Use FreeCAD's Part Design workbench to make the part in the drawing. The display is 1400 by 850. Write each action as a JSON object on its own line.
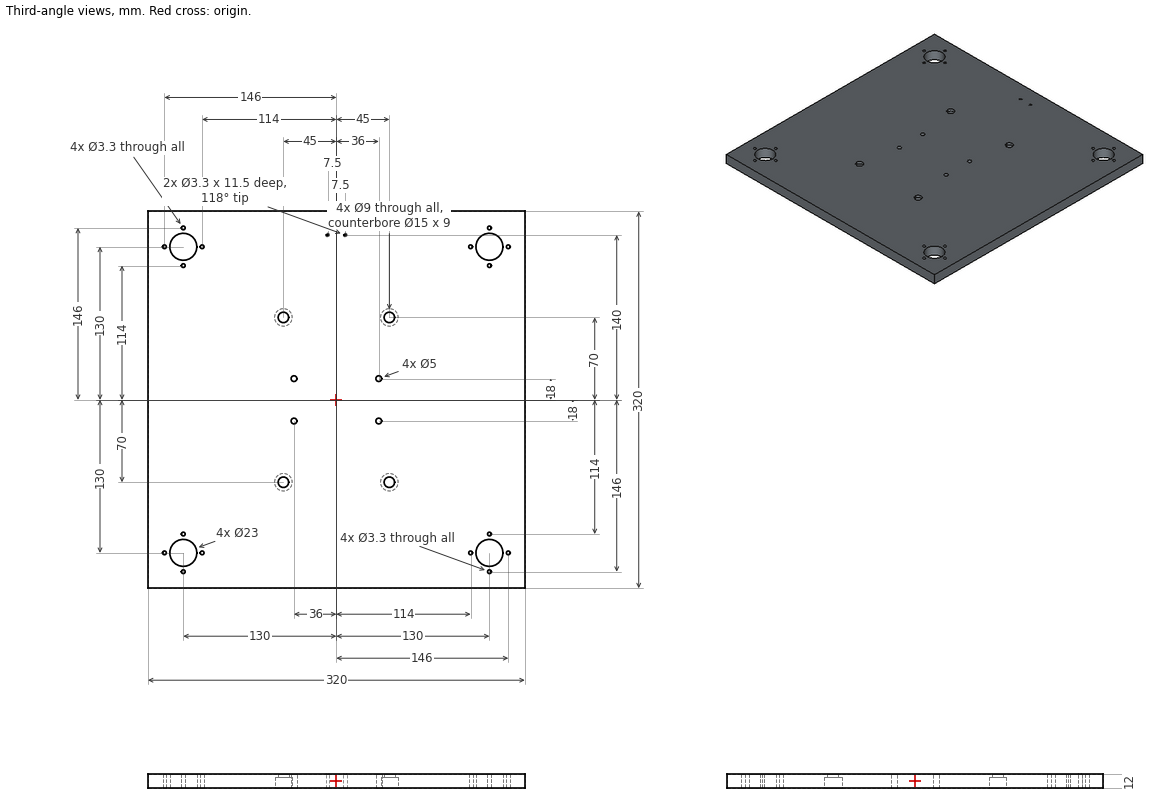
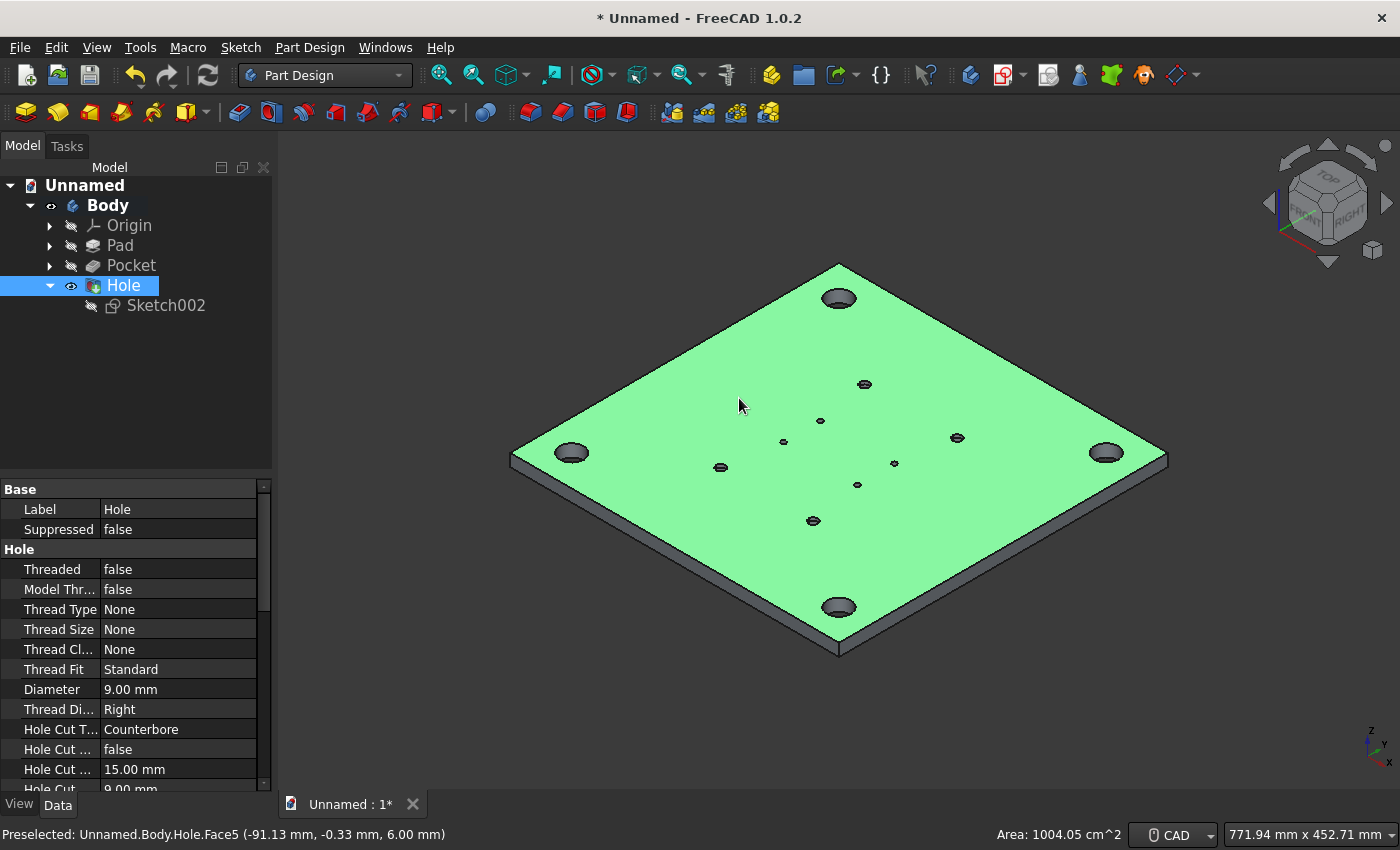
{"action": "left_click", "coordinate": [1004, 76]}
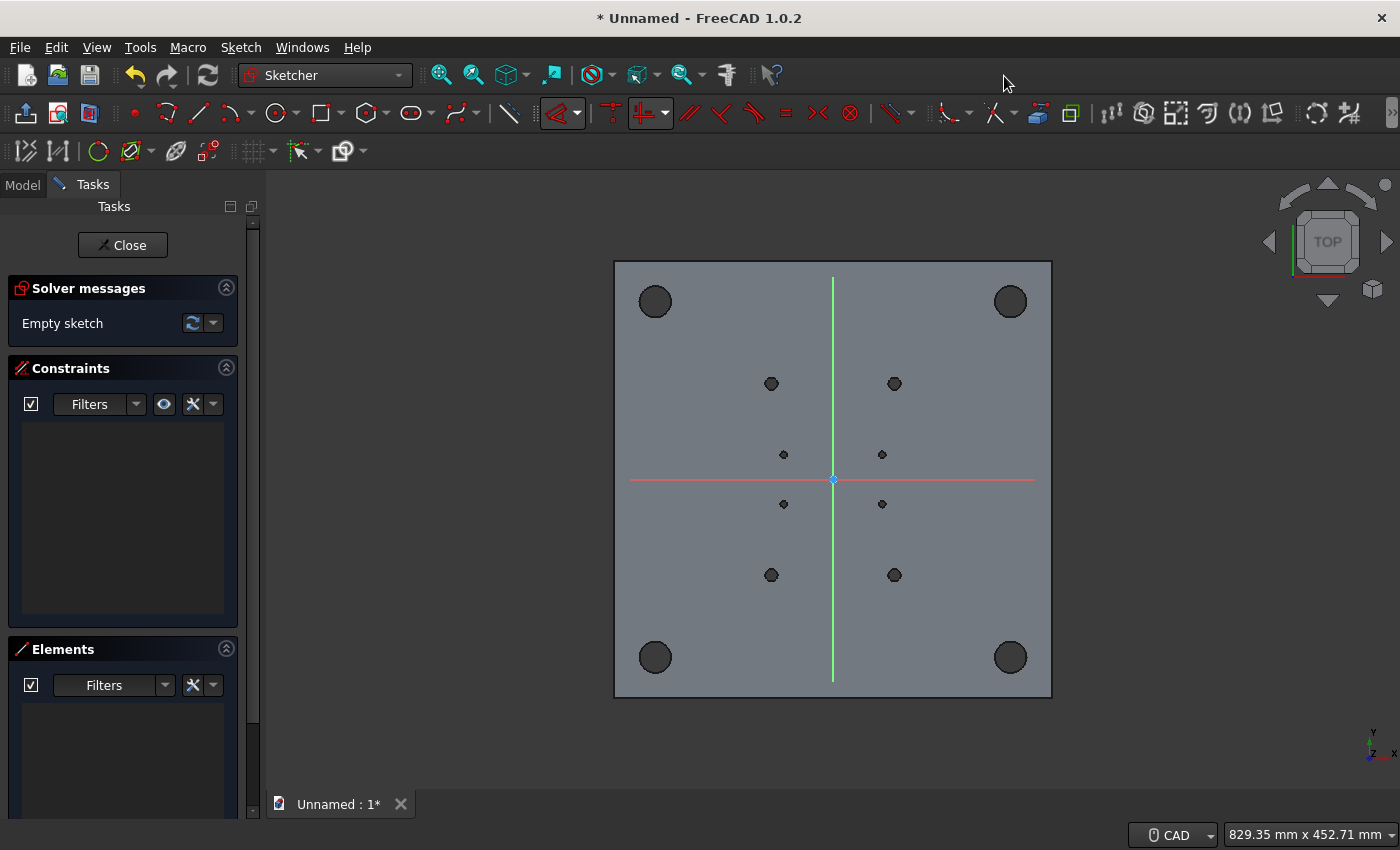
{"action": "scroll", "coordinate": [642, 280], "scroll_direction": "up", "scroll_amount": 11}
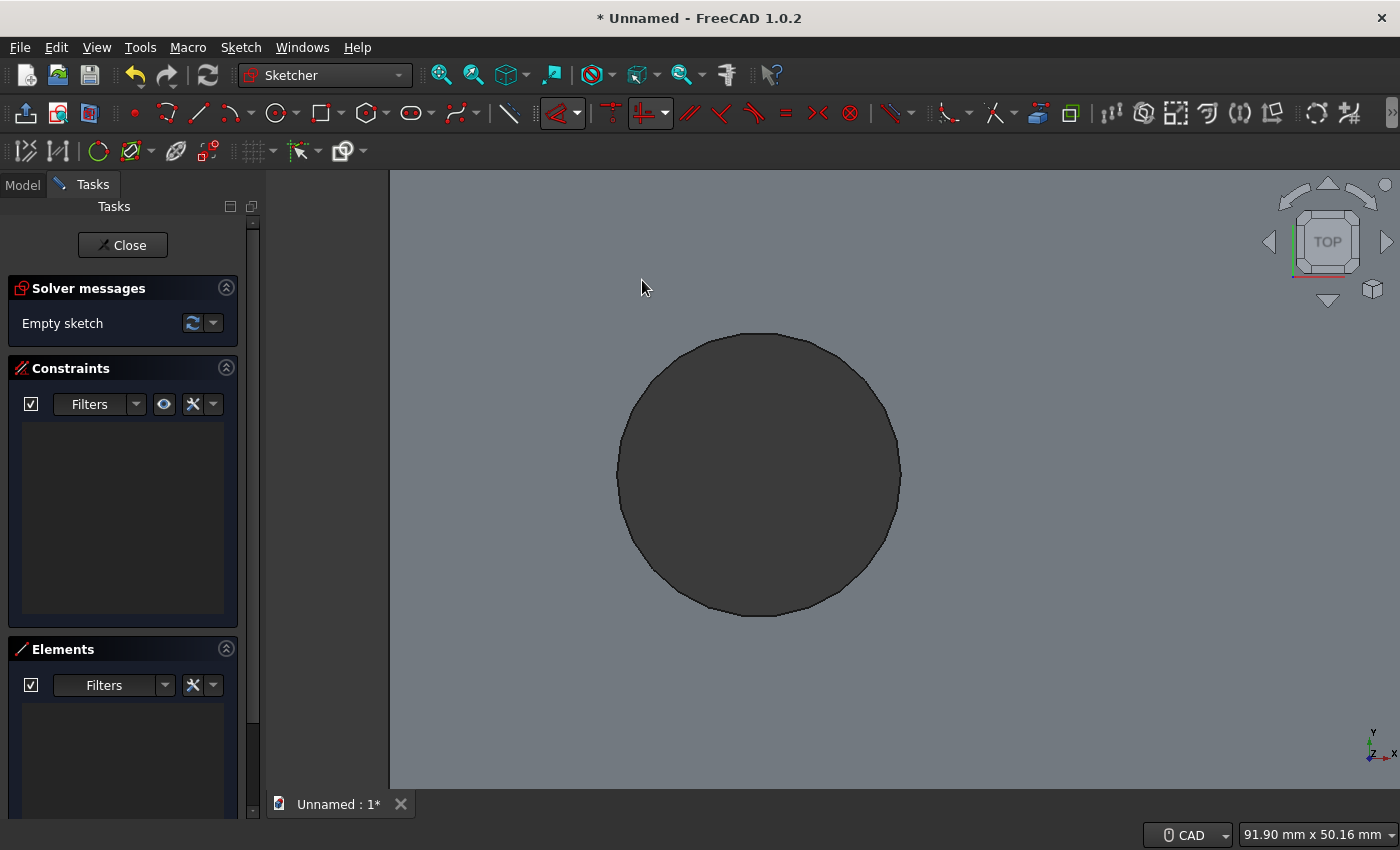
{"action": "left_click", "coordinate": [276, 114]}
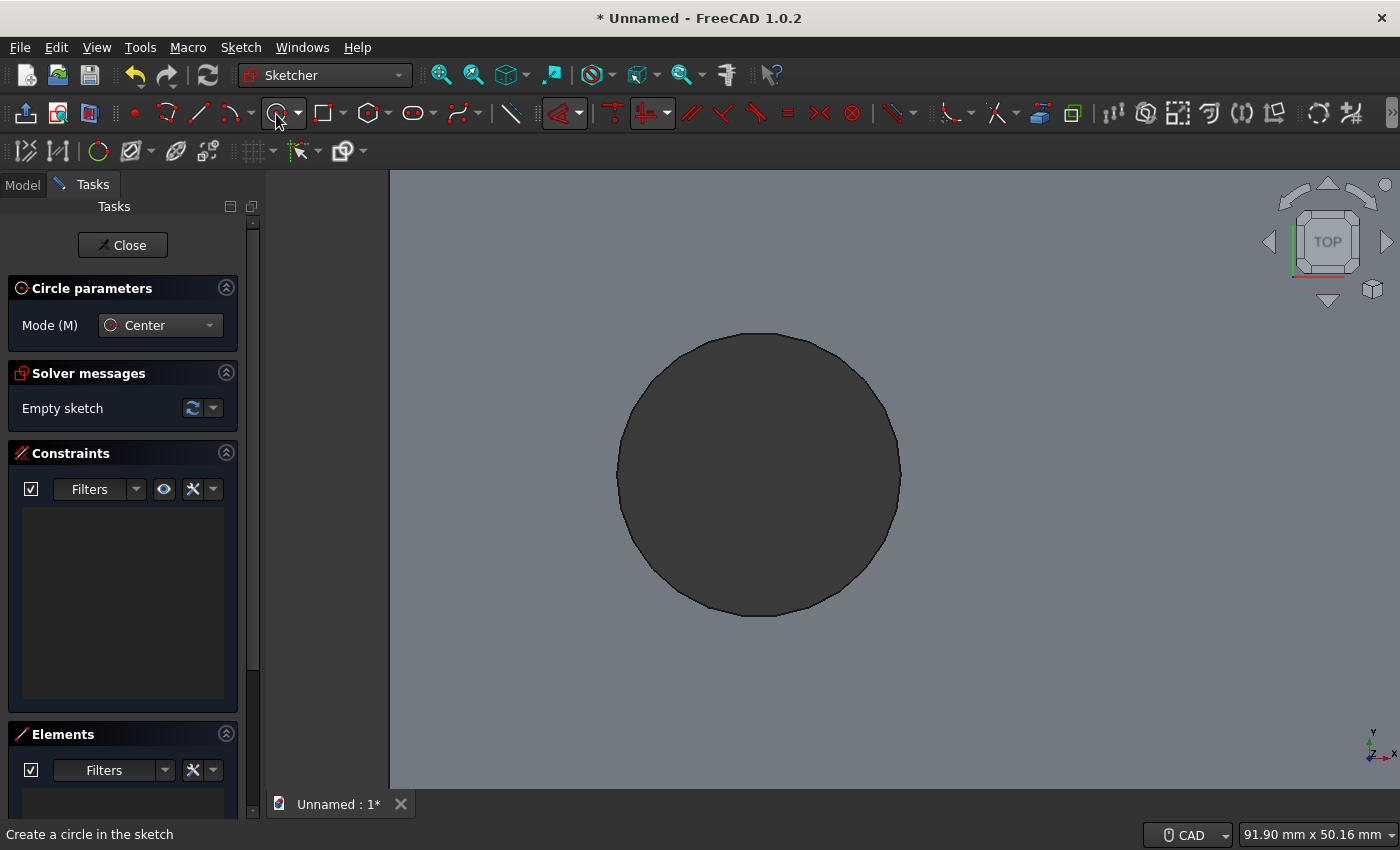
{"action": "left_click", "coordinate": [759, 277]}
{"action": "mouse_move", "coordinate": [773, 263]}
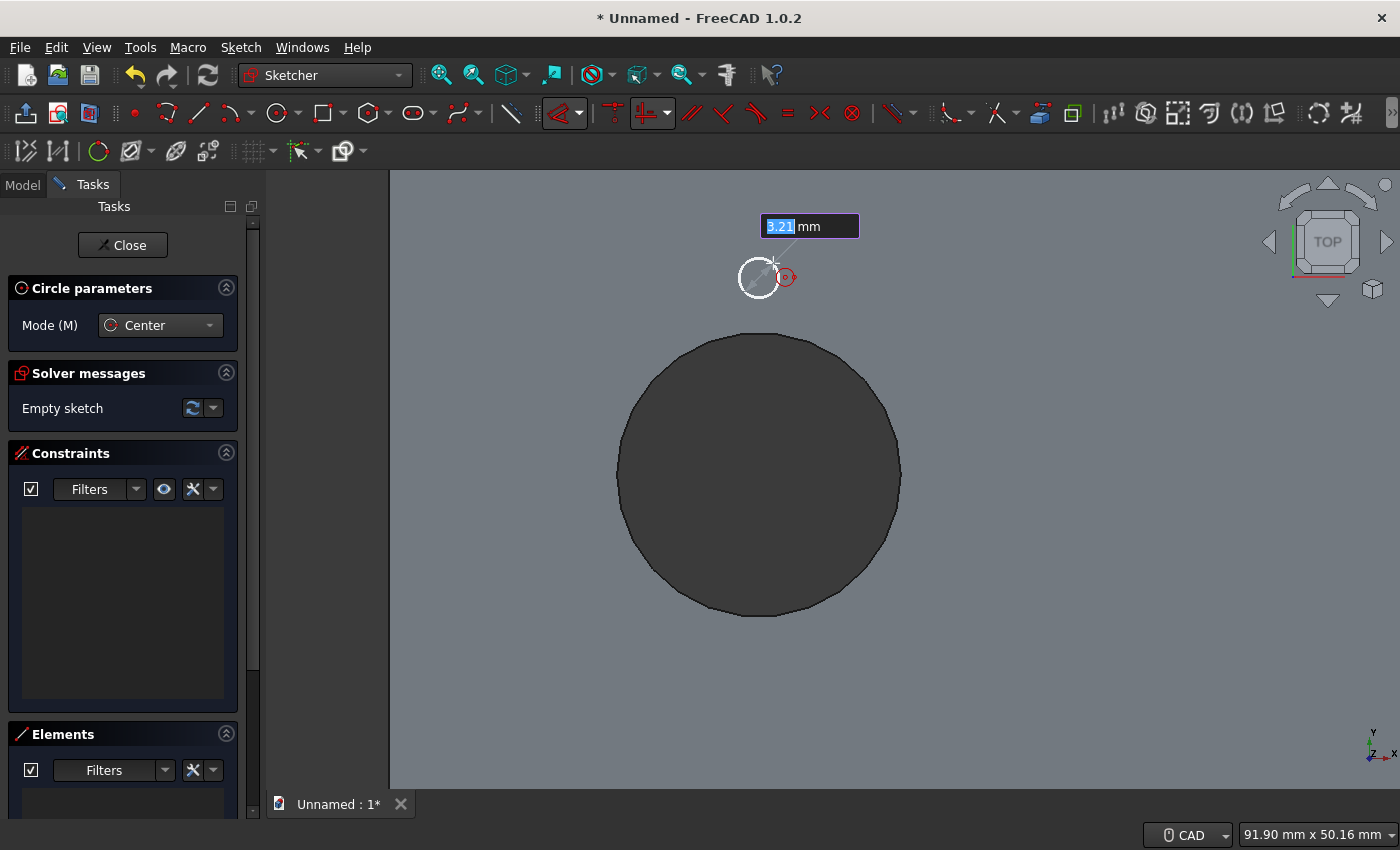
{"action": "type", "text": "3.3"}
{"action": "key", "text": "Return"}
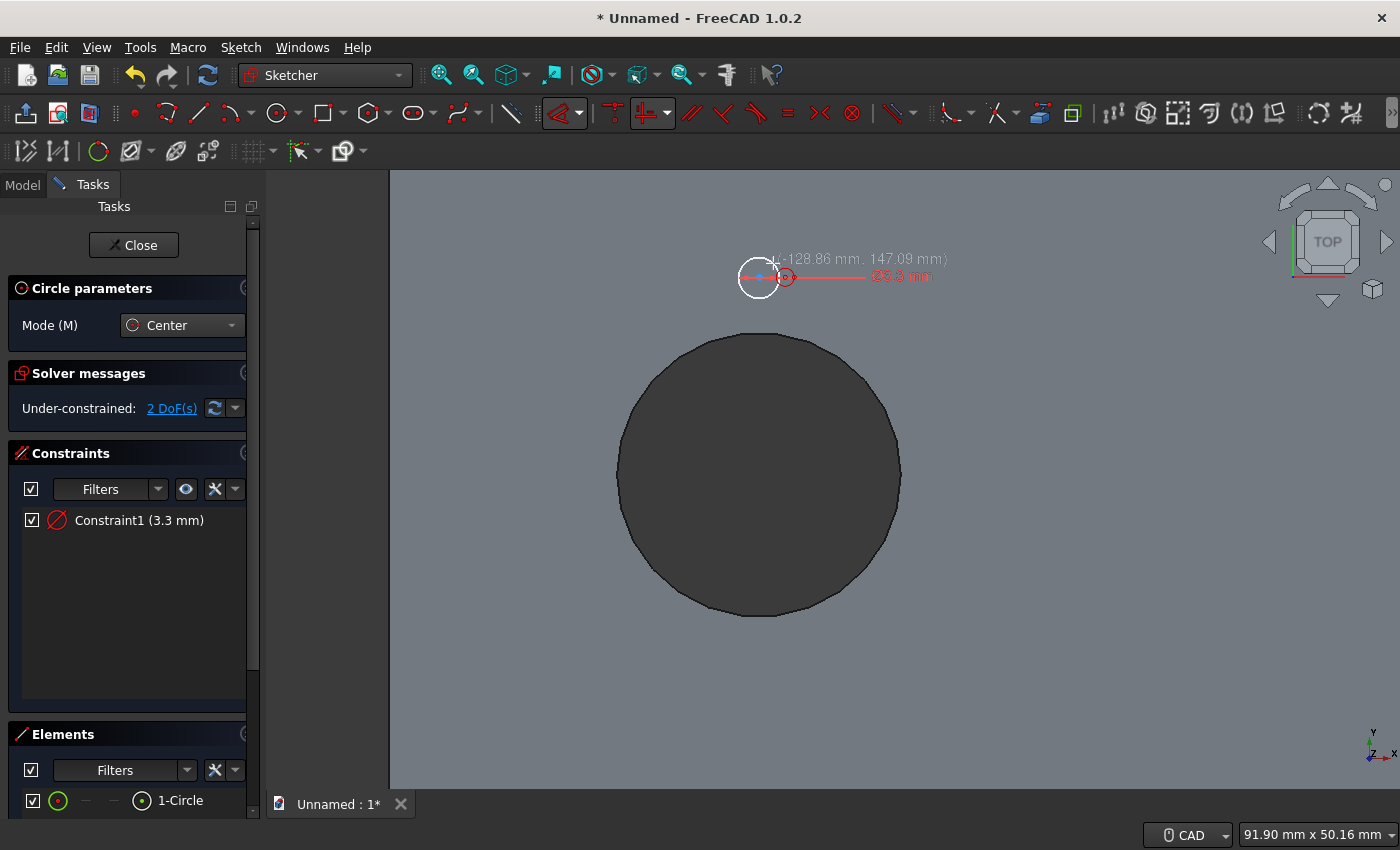
{"action": "left_click", "coordinate": [956, 475]}
{"action": "mouse_move", "coordinate": [971, 460]}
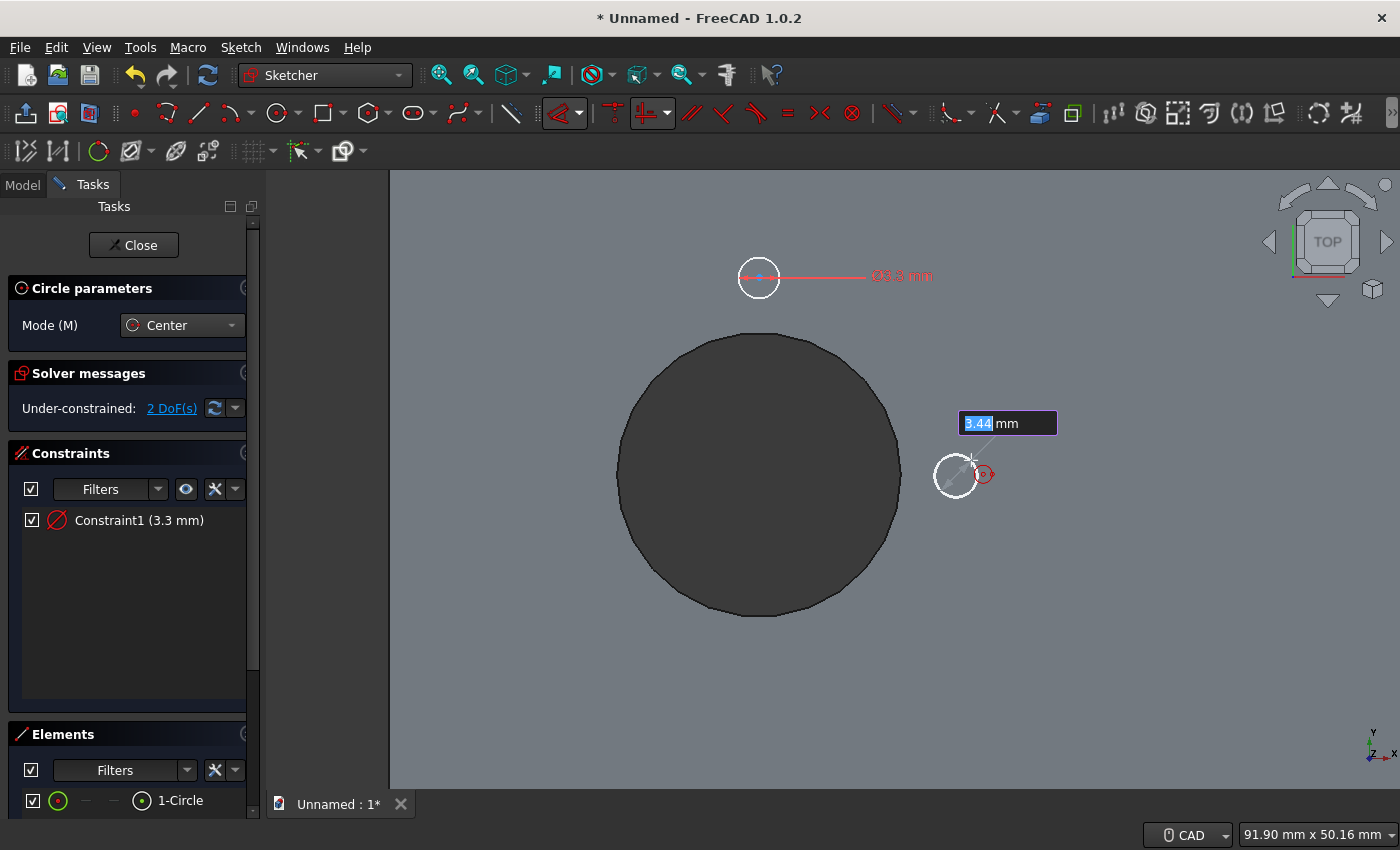
{"action": "type", "text": "3.3"}
{"action": "key", "text": "Return"}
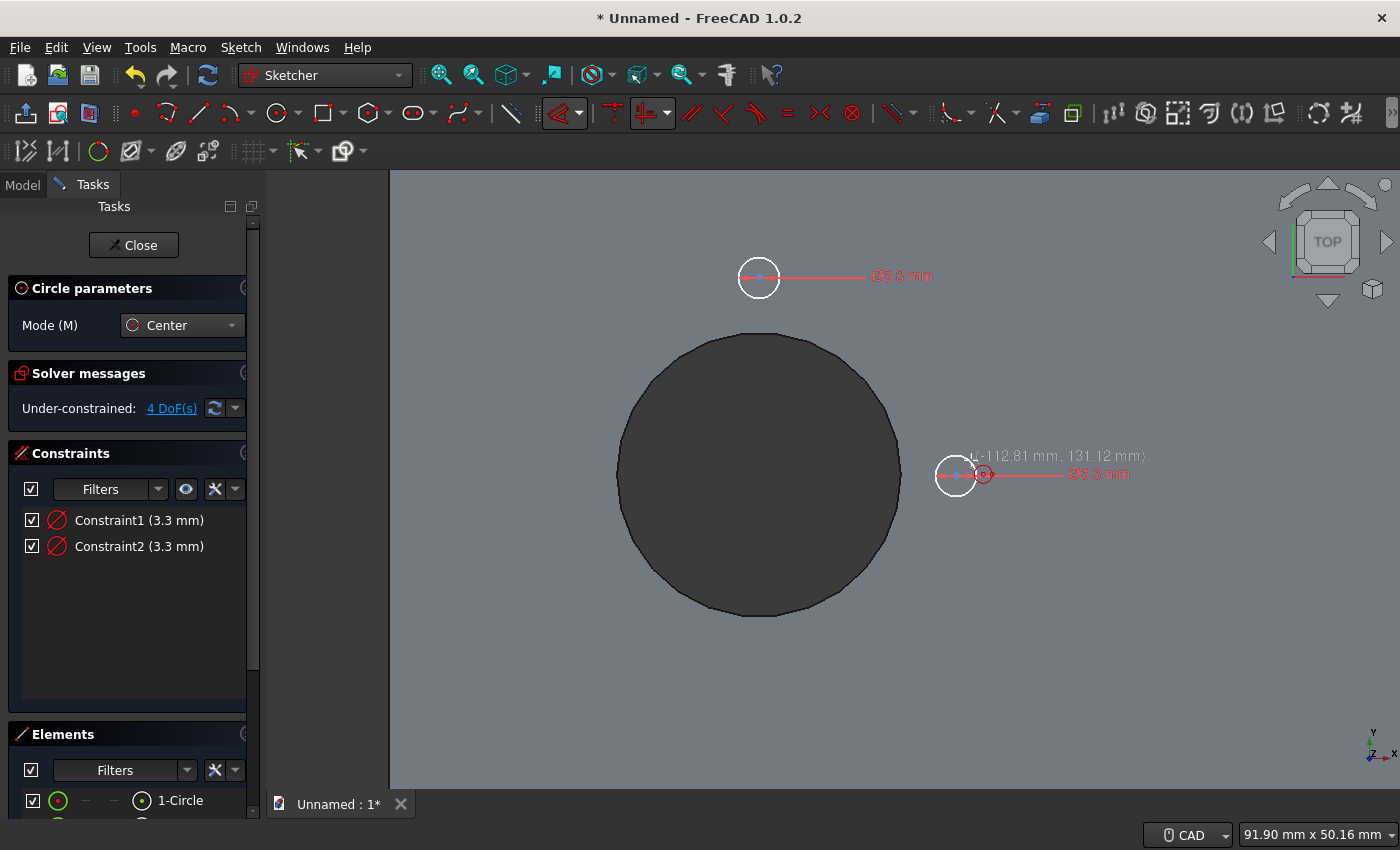
{"action": "left_click", "coordinate": [759, 672]}
{"action": "mouse_move", "coordinate": [773, 658]}